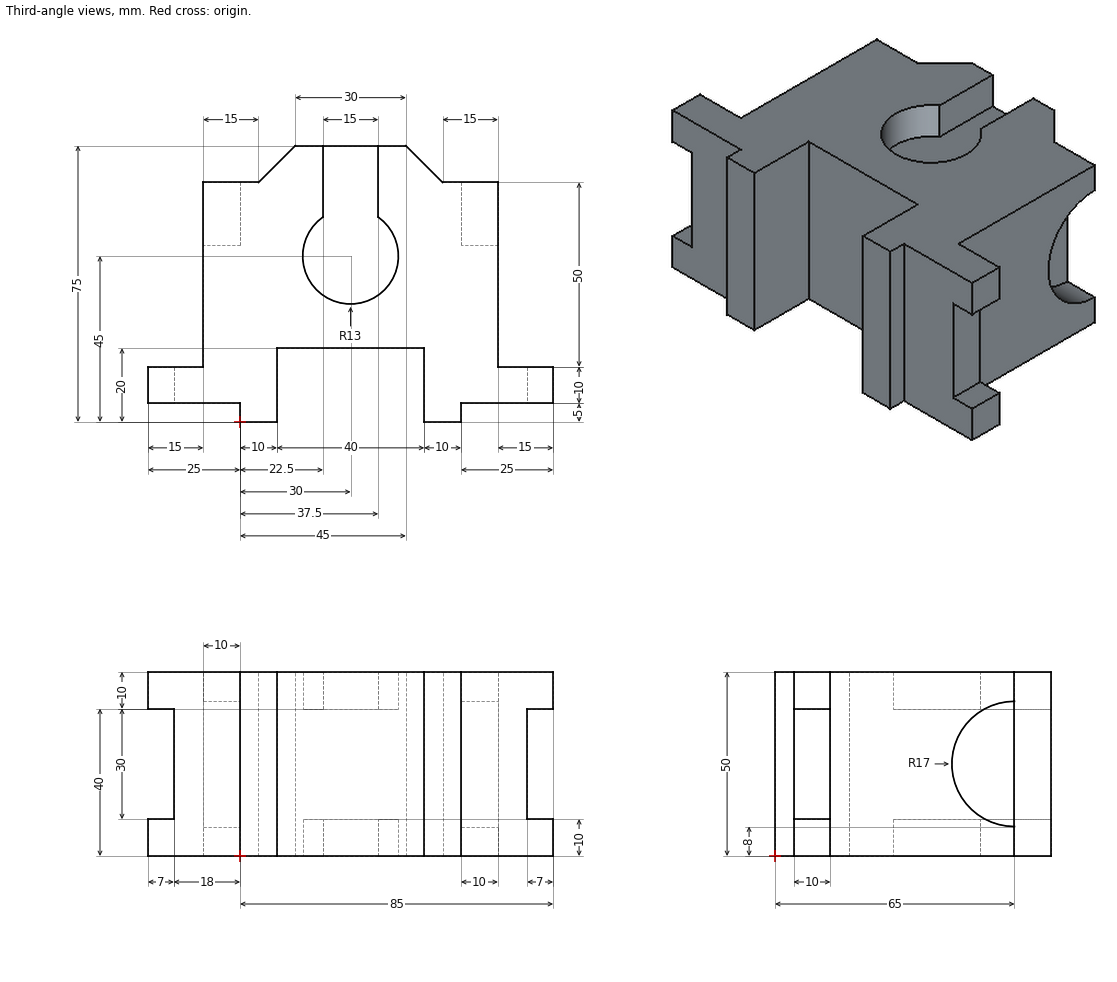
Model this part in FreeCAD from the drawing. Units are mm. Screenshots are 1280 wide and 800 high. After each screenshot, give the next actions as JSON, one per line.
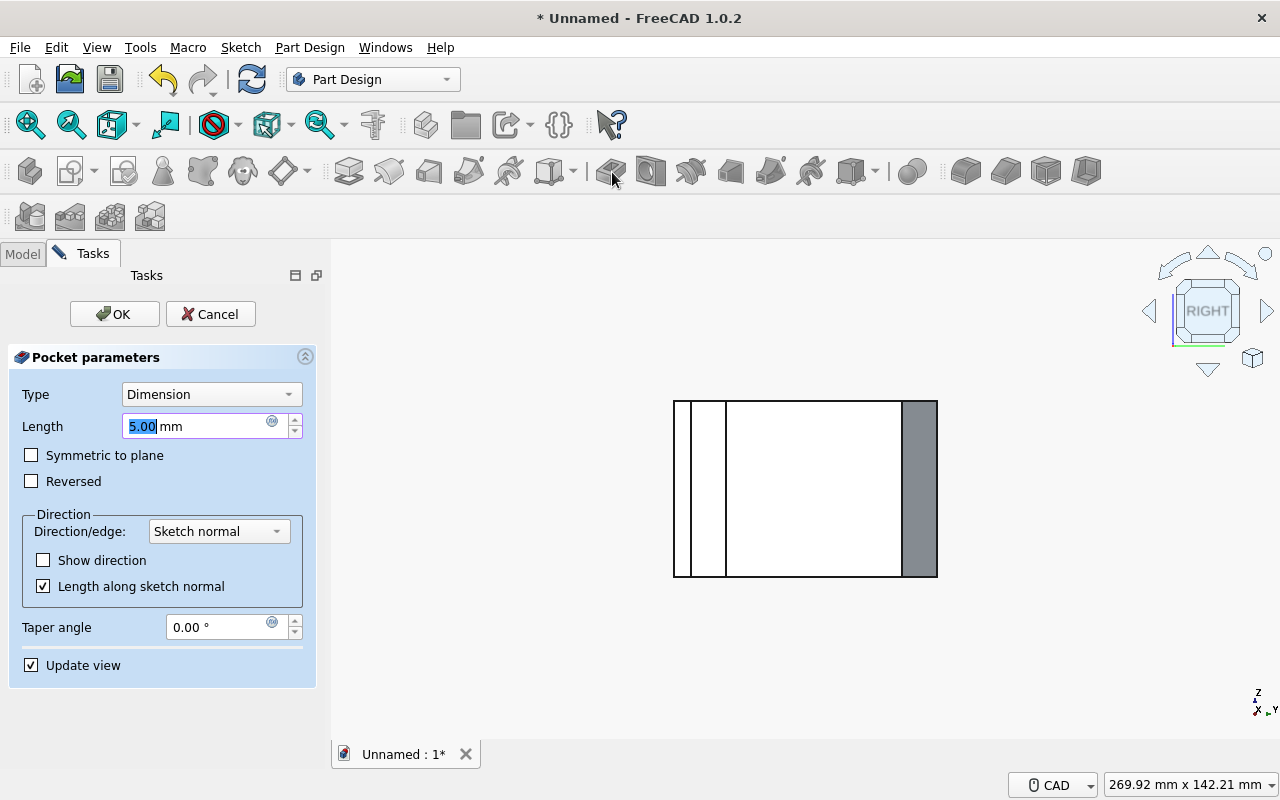
{"action": "type", "text": "10"}
{"action": "key", "text": "Tab"}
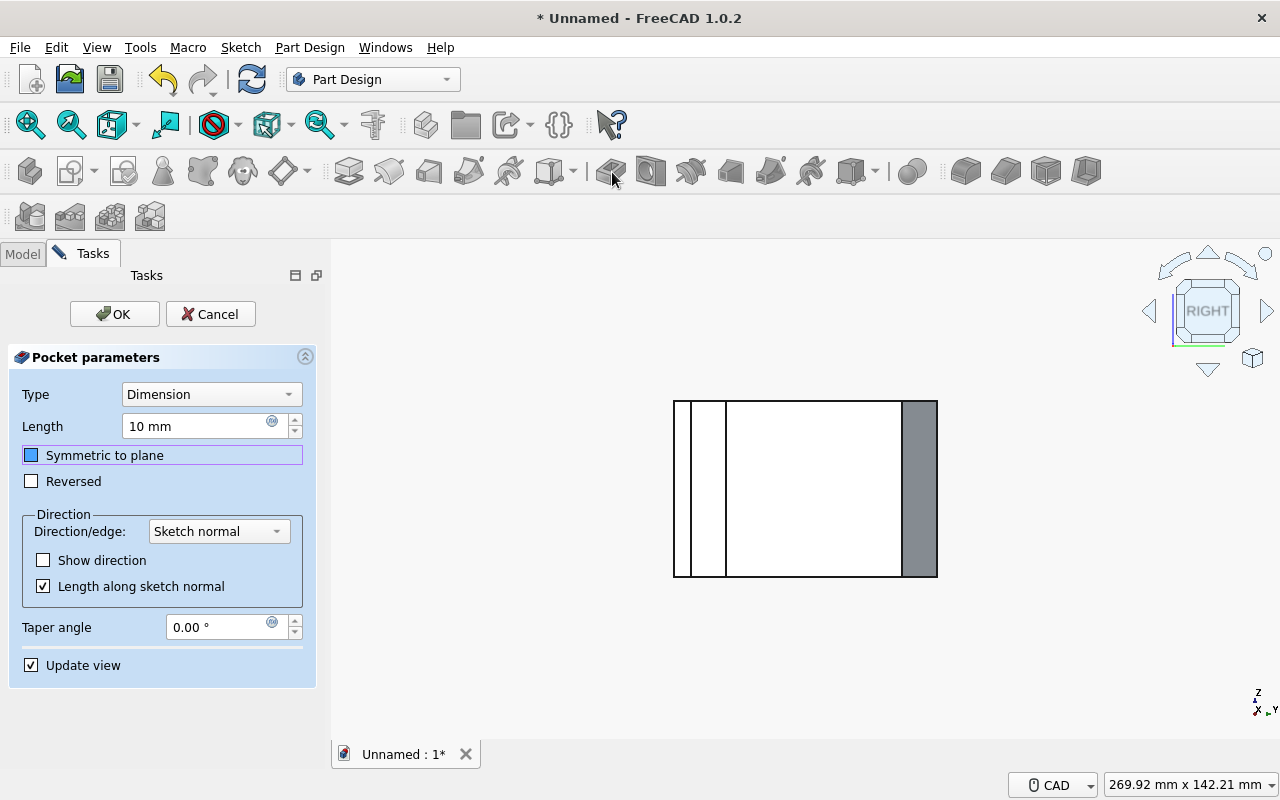
{"action": "left_click", "coordinate": [30, 481]}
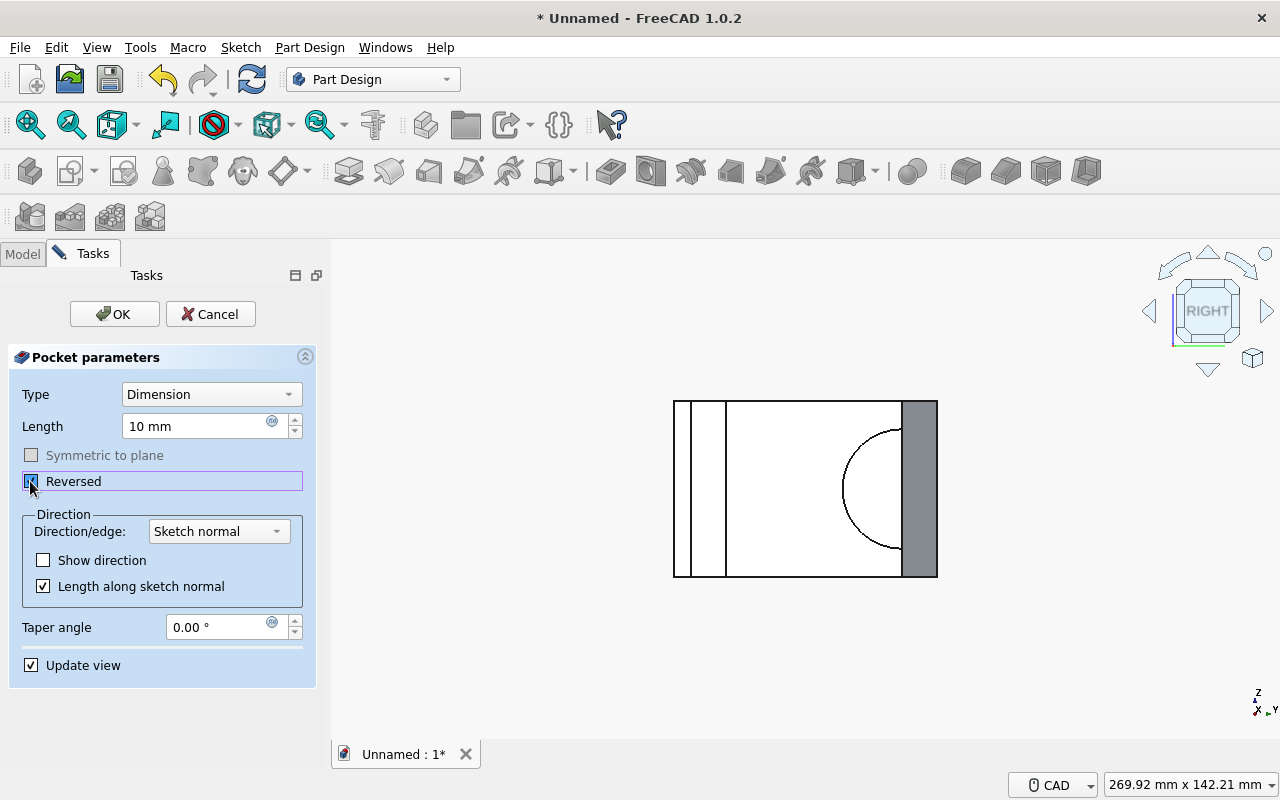
{"action": "left_click", "coordinate": [115, 314]}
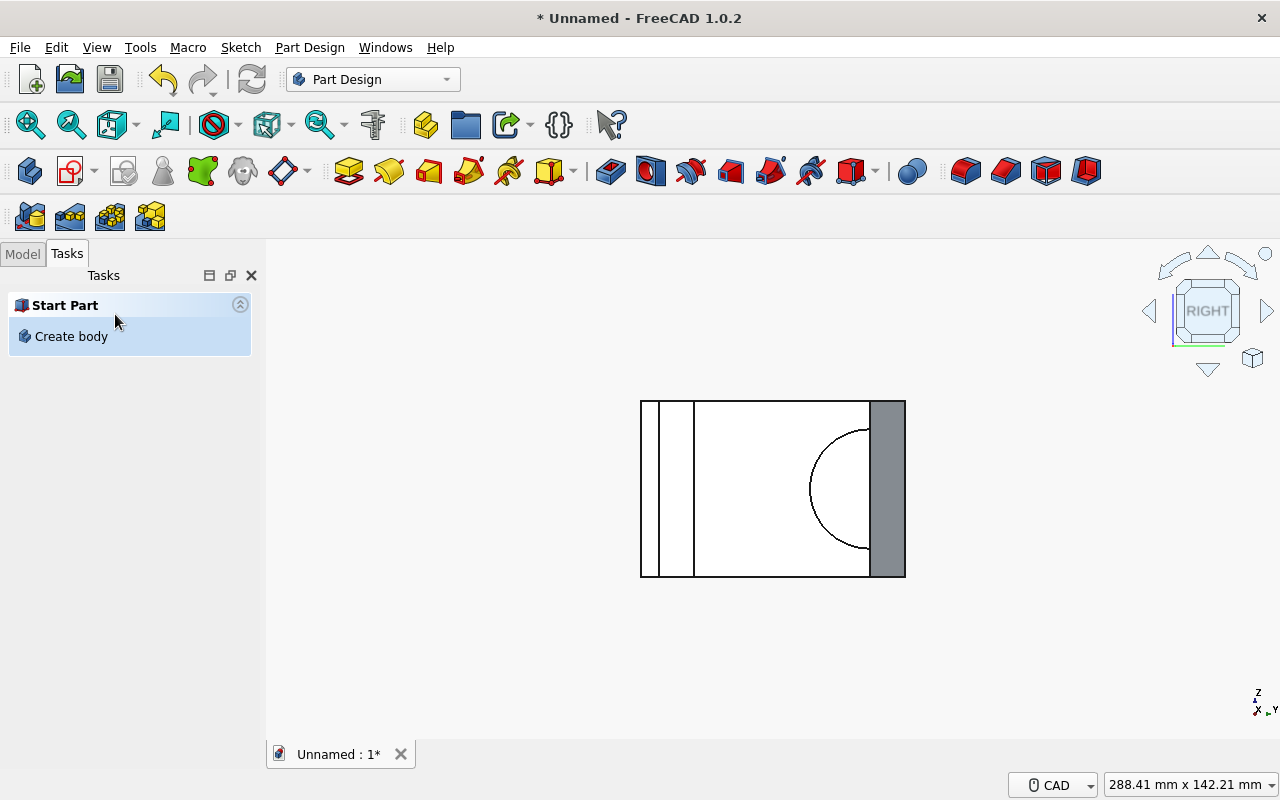
{"action": "left_click", "coordinate": [32, 126]}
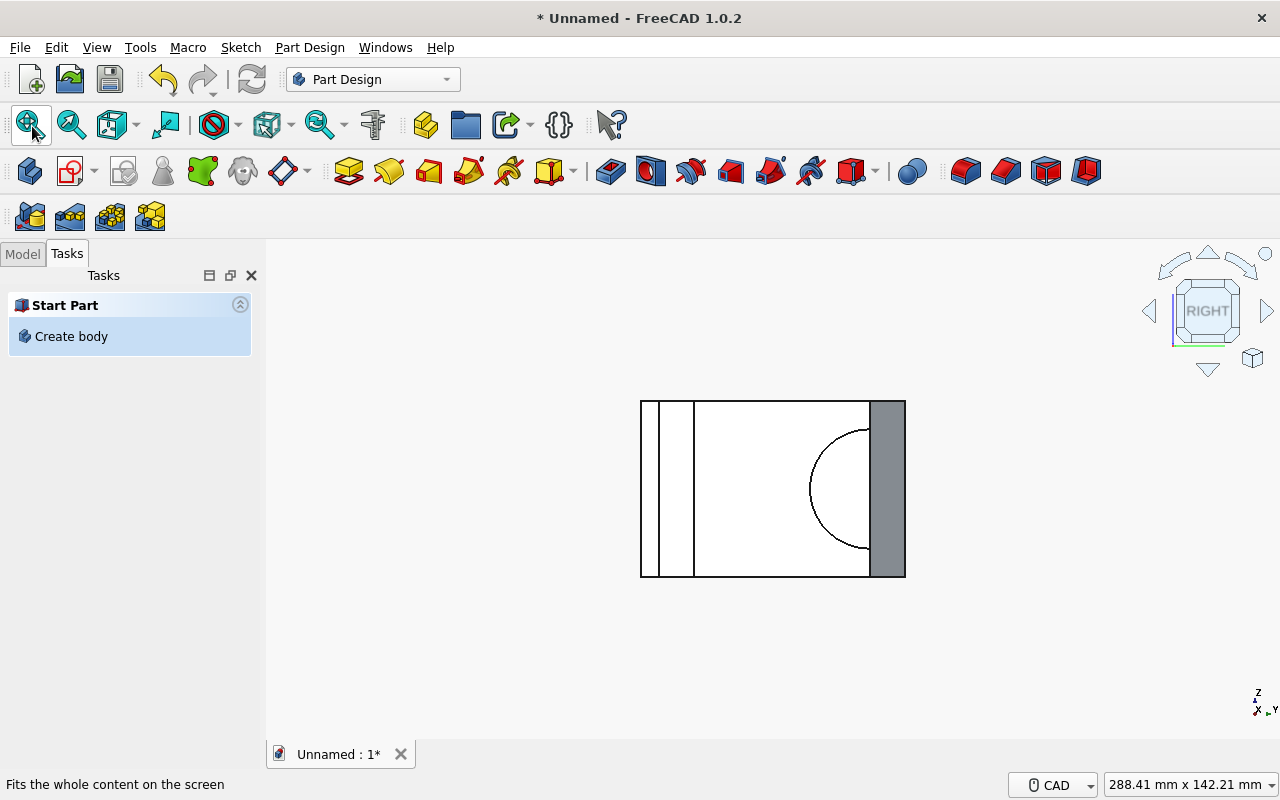
{"action": "key", "text": "5"}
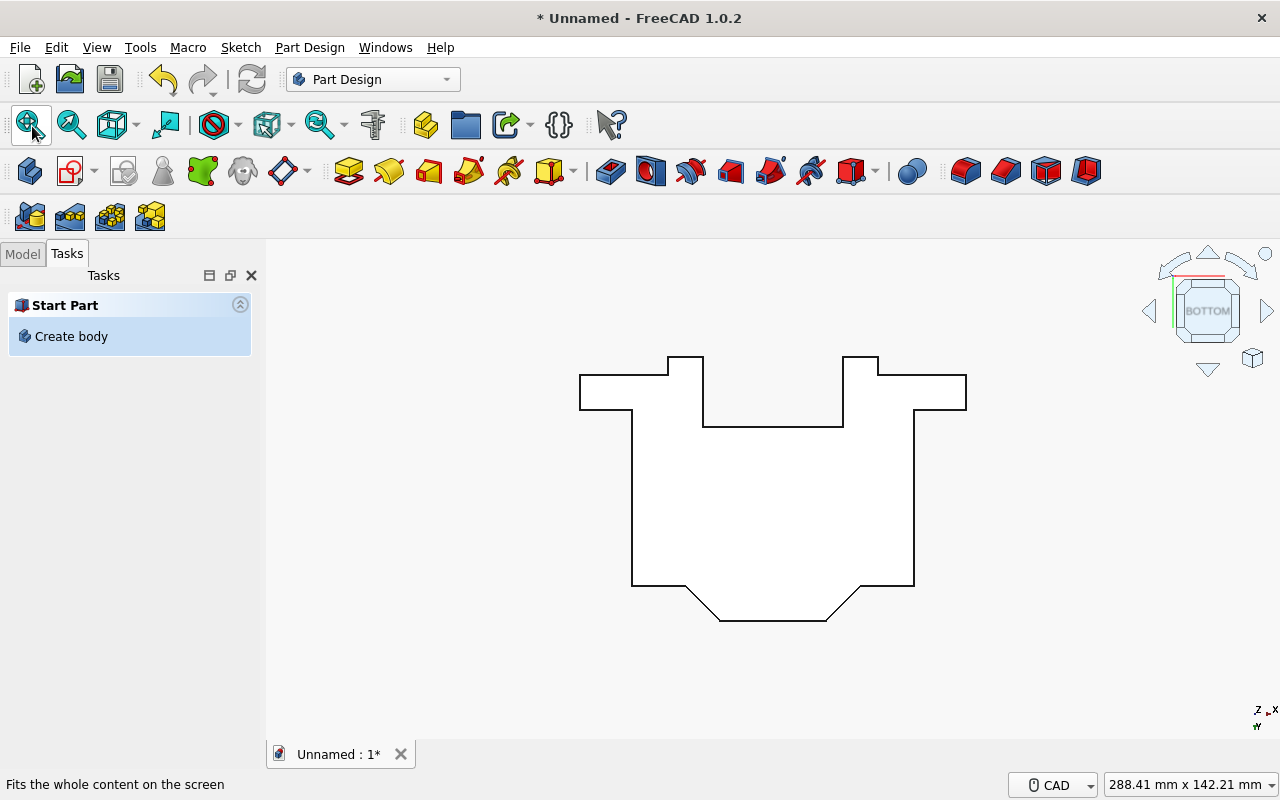
{"action": "left_click", "coordinate": [773, 526]}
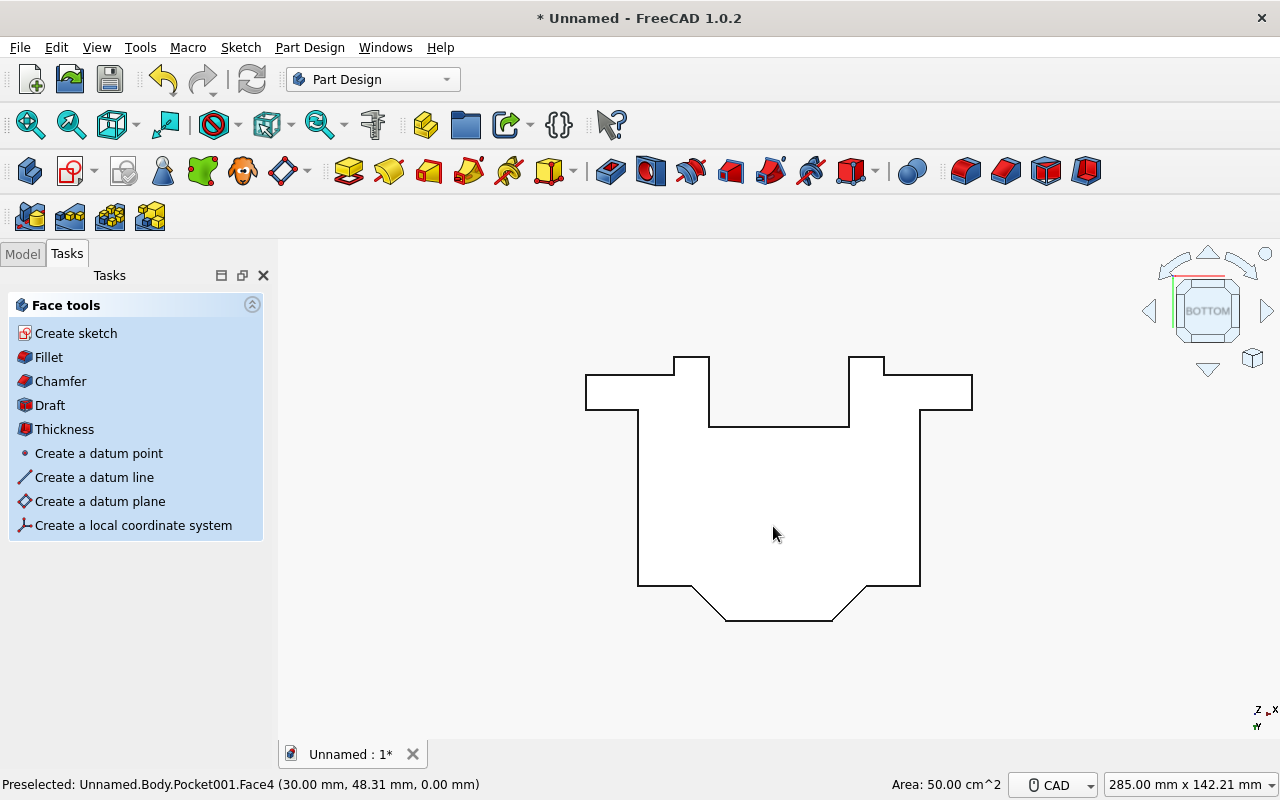
{"action": "left_click", "coordinate": [70, 172]}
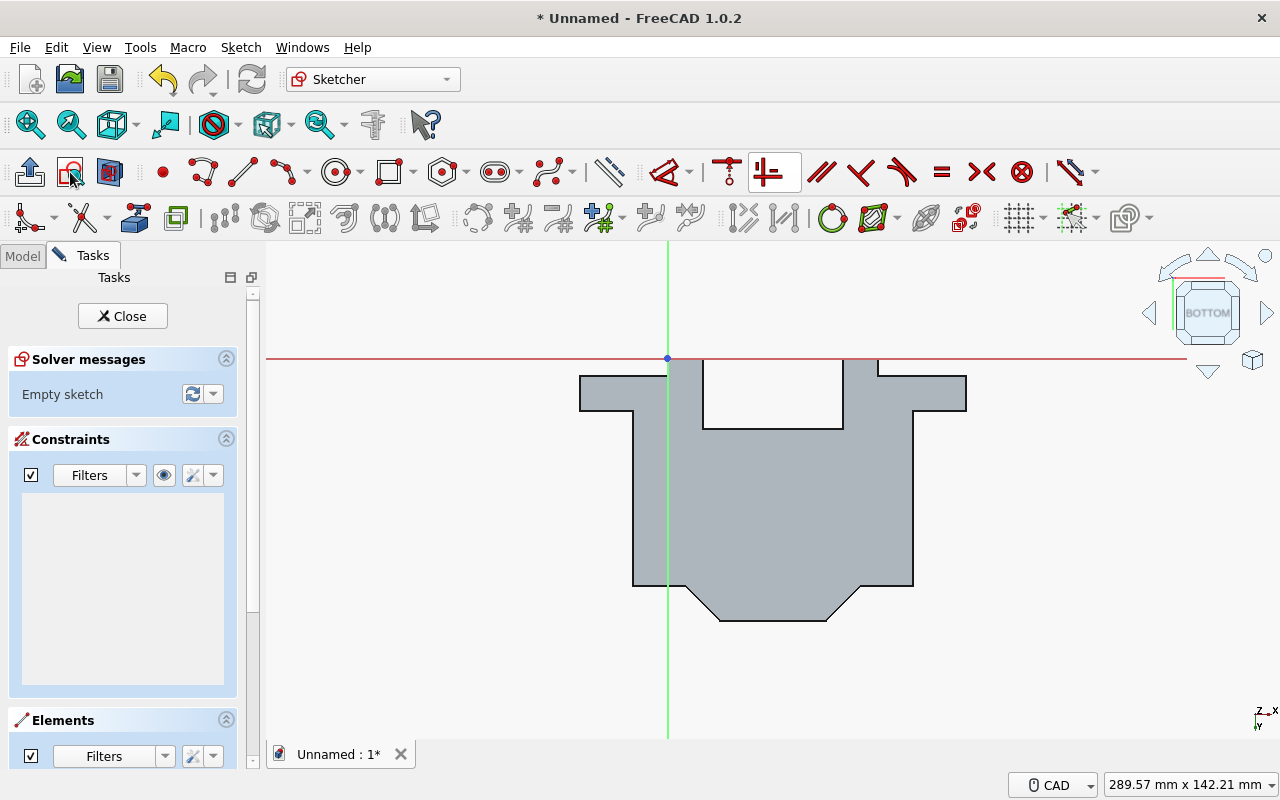
{"action": "left_click", "coordinate": [204, 172]}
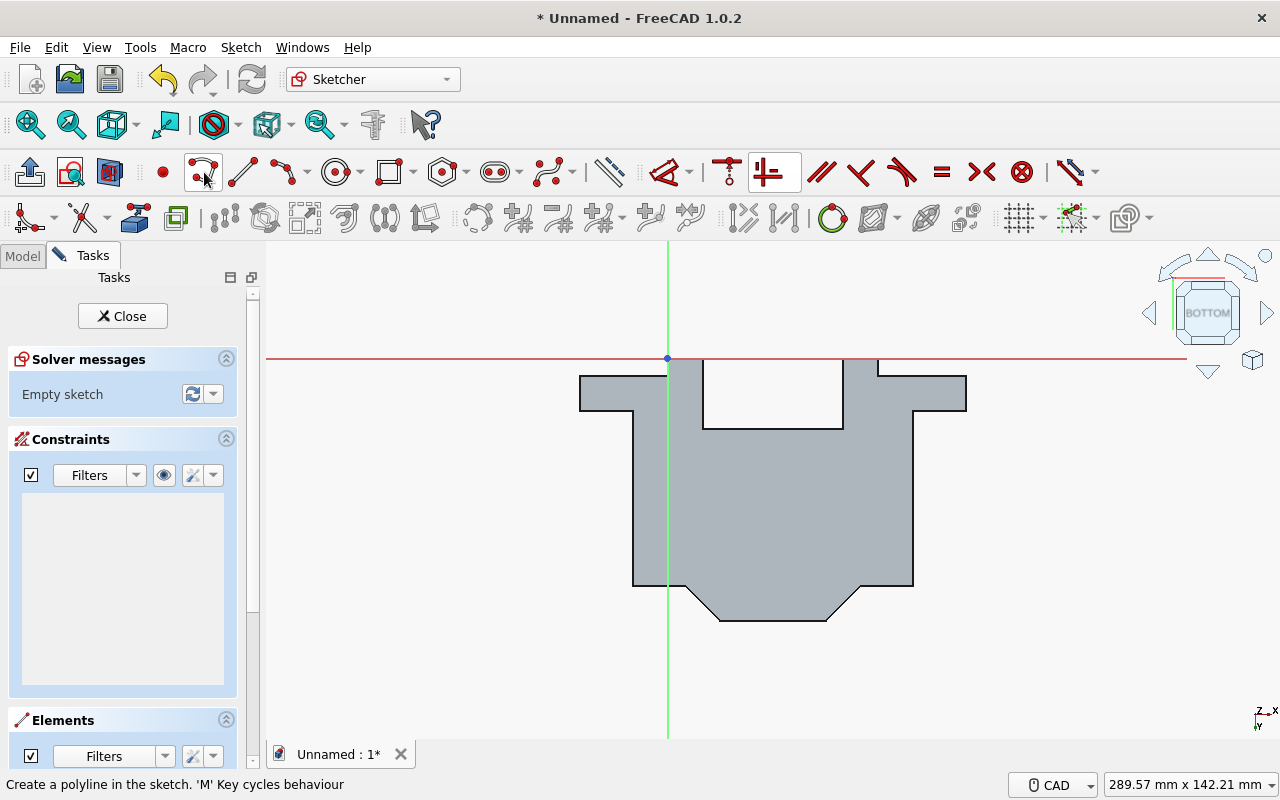
{"action": "left_click", "coordinate": [747, 553]}
{"action": "left_click", "coordinate": [747, 621]}
{"action": "left_click", "coordinate": [799, 621]}
{"action": "left_click", "coordinate": [799, 553]}
{"action": "right_click", "coordinate": [799, 553]}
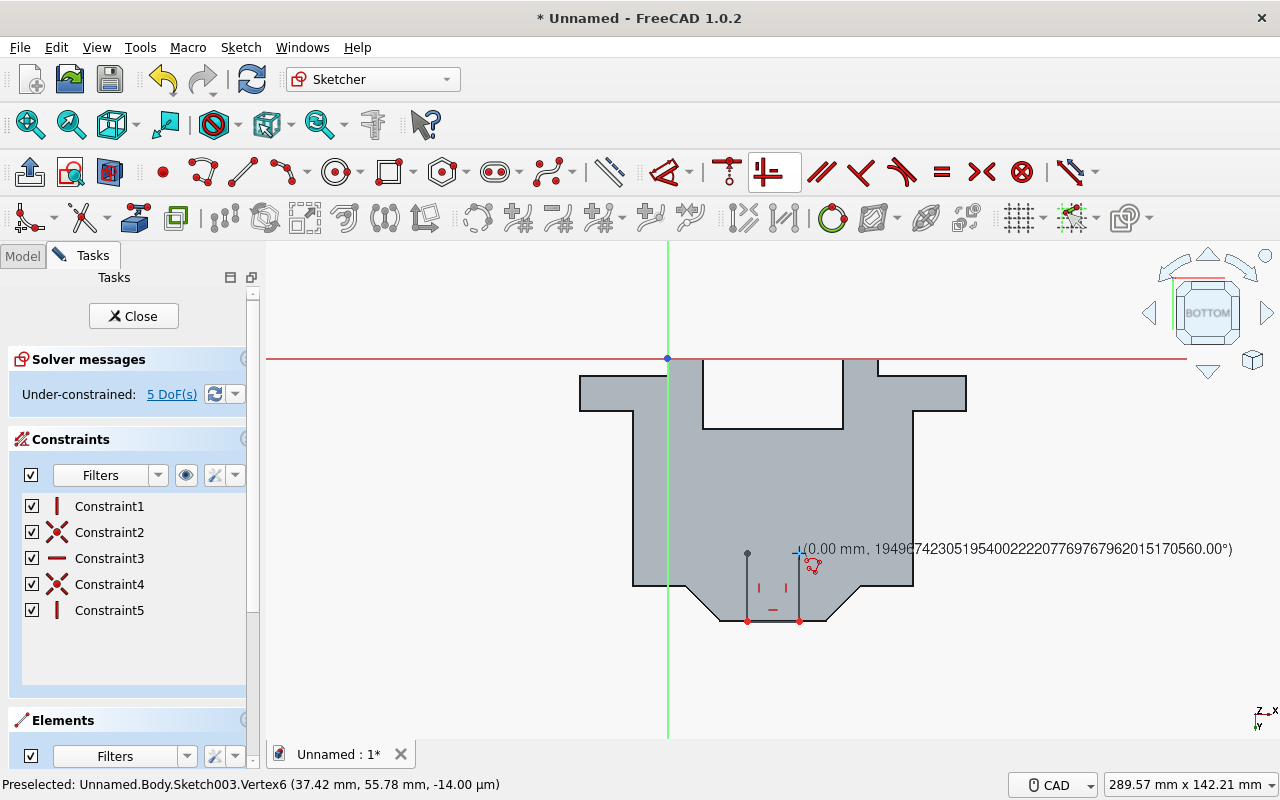
{"action": "left_click", "coordinate": [284, 172]}